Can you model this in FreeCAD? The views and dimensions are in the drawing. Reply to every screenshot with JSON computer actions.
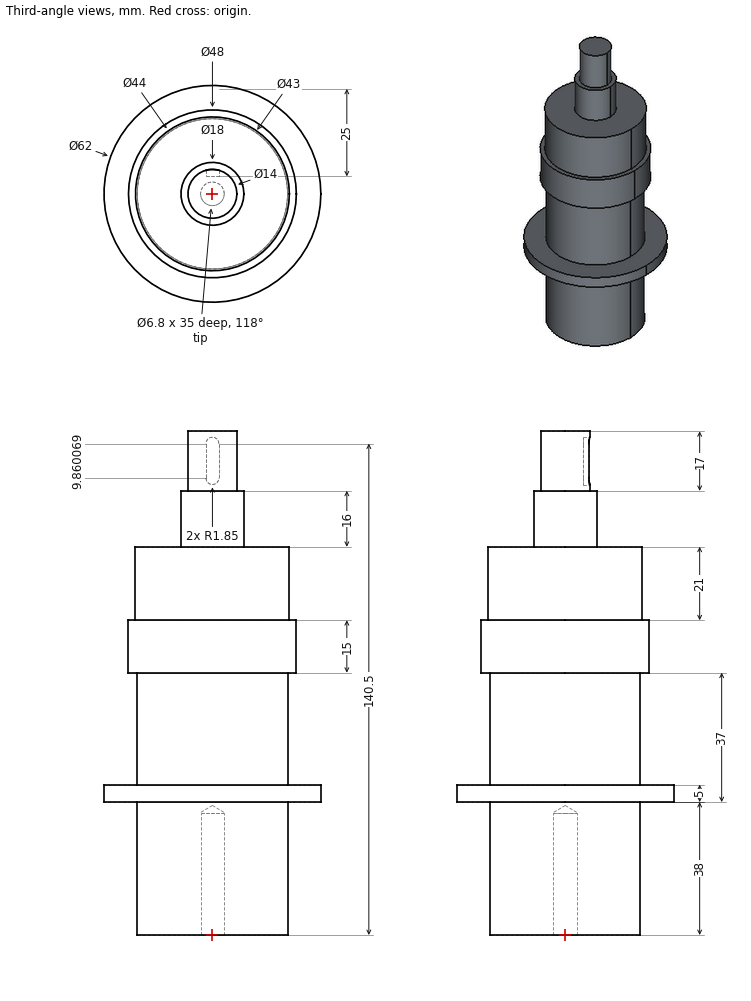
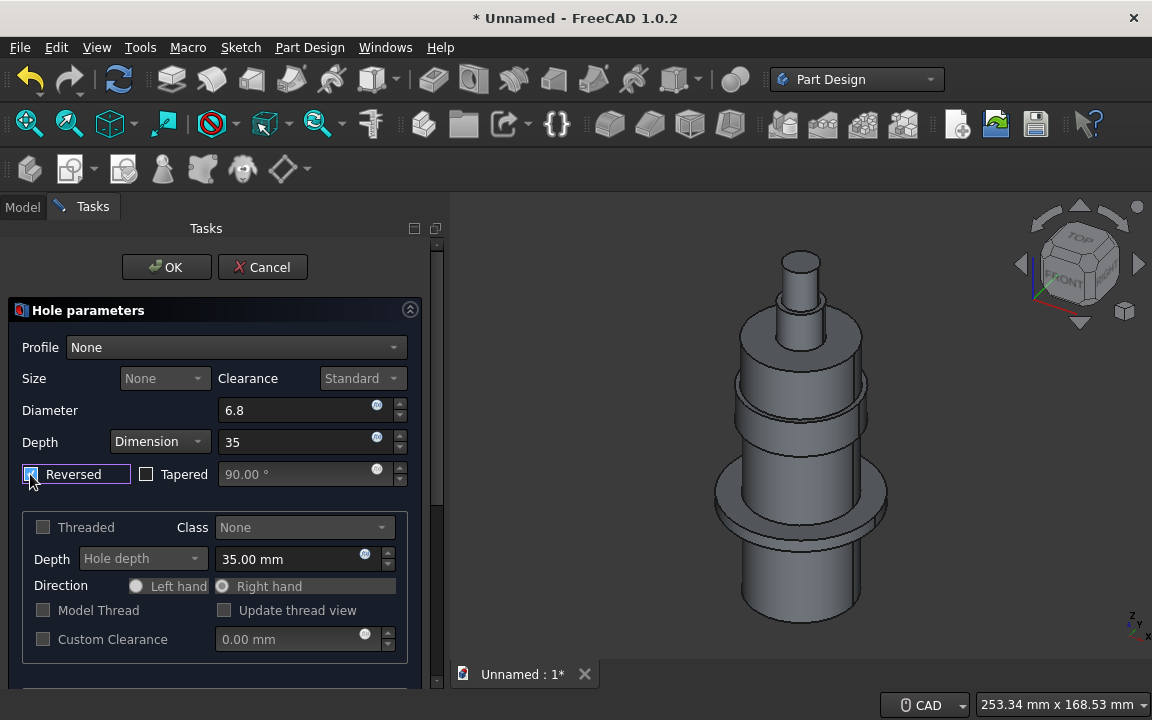
{"action": "left_click", "coordinate": [167, 267]}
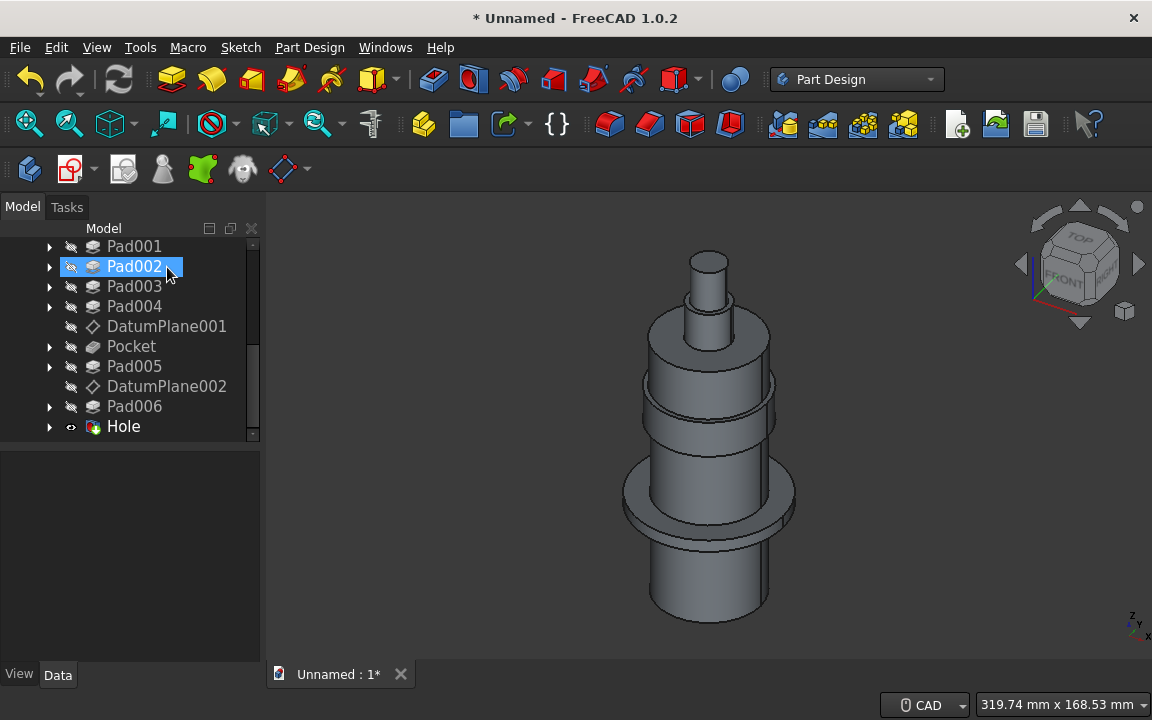
{"action": "key", "text": "0"}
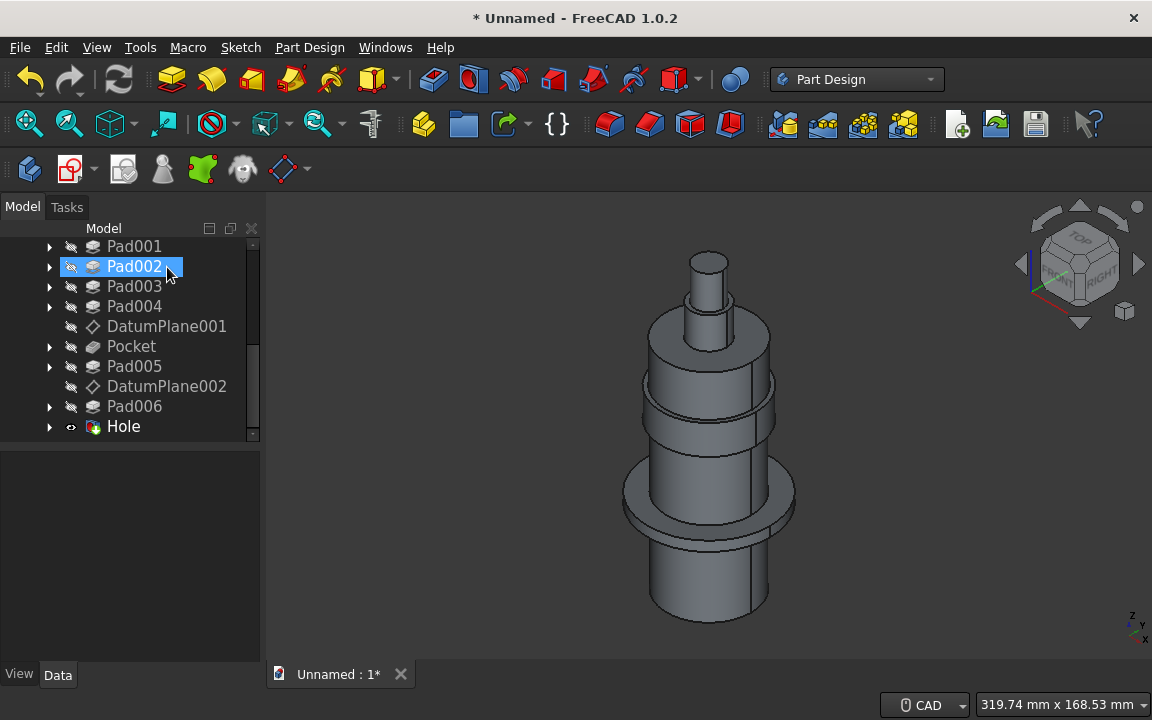
{"action": "key", "text": "v f"}